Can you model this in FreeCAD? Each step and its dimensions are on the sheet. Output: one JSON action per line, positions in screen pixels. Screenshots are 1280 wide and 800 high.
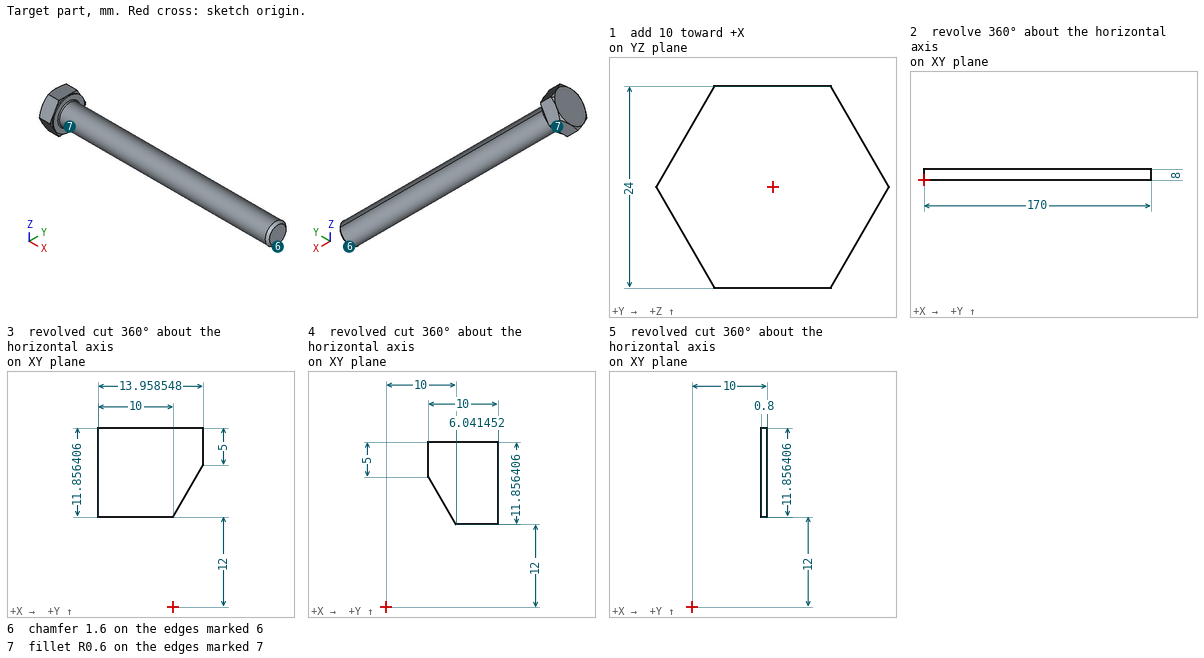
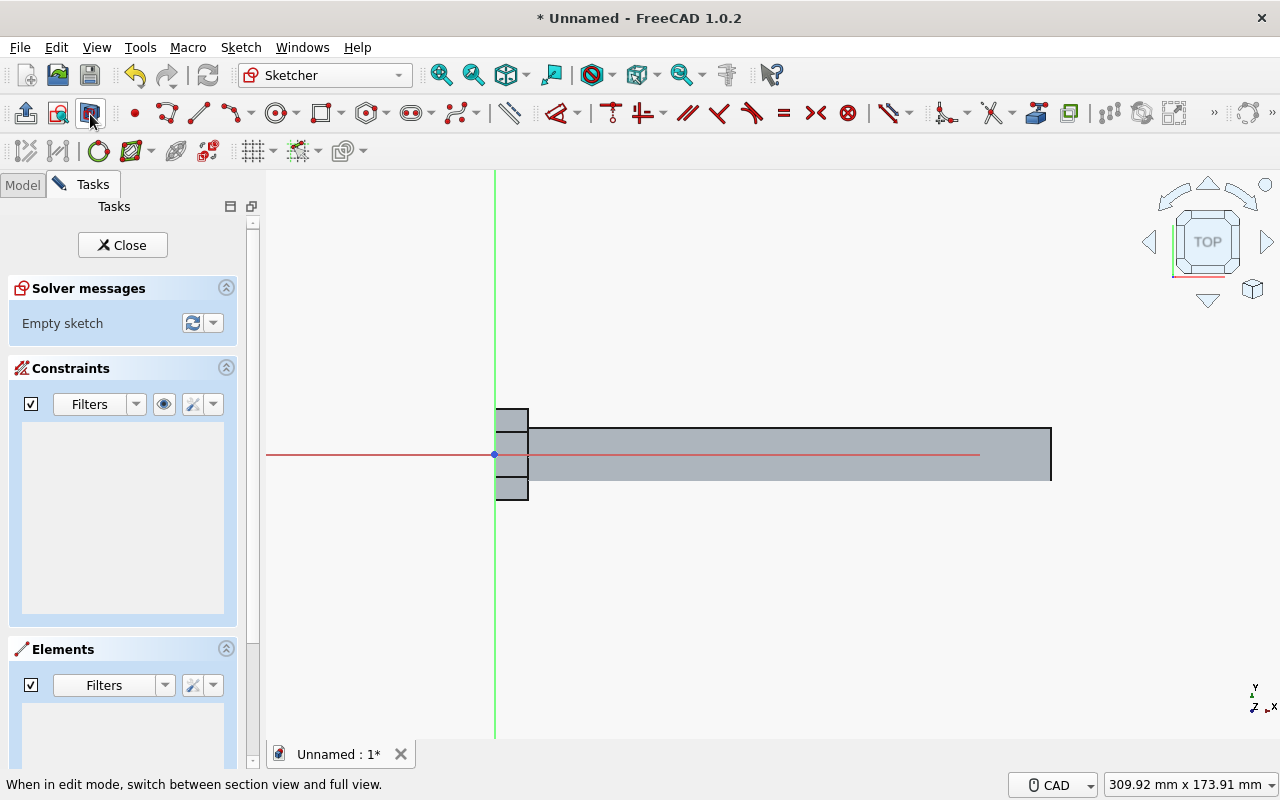
{"action": "scroll", "coordinate": [429, 406], "scroll_direction": "up", "scroll_amount": 8}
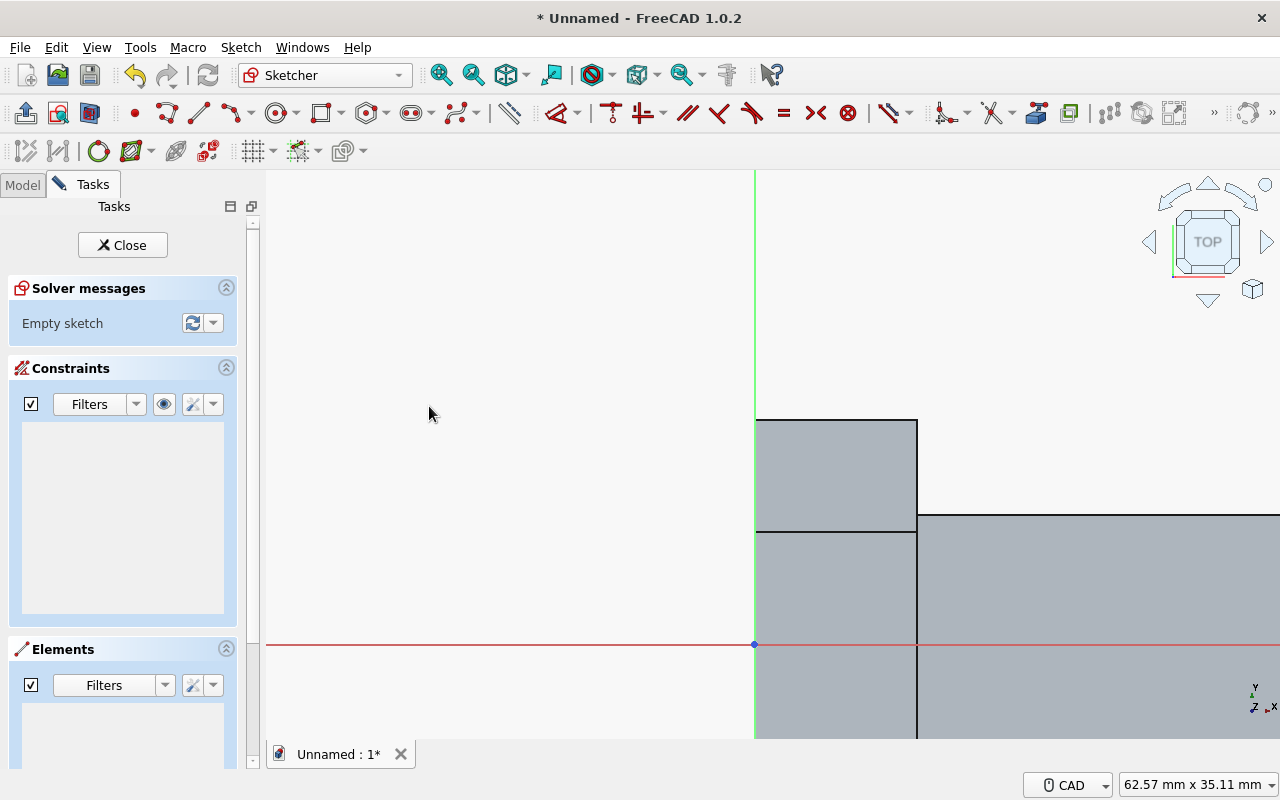
{"action": "left_click", "coordinate": [168, 114]}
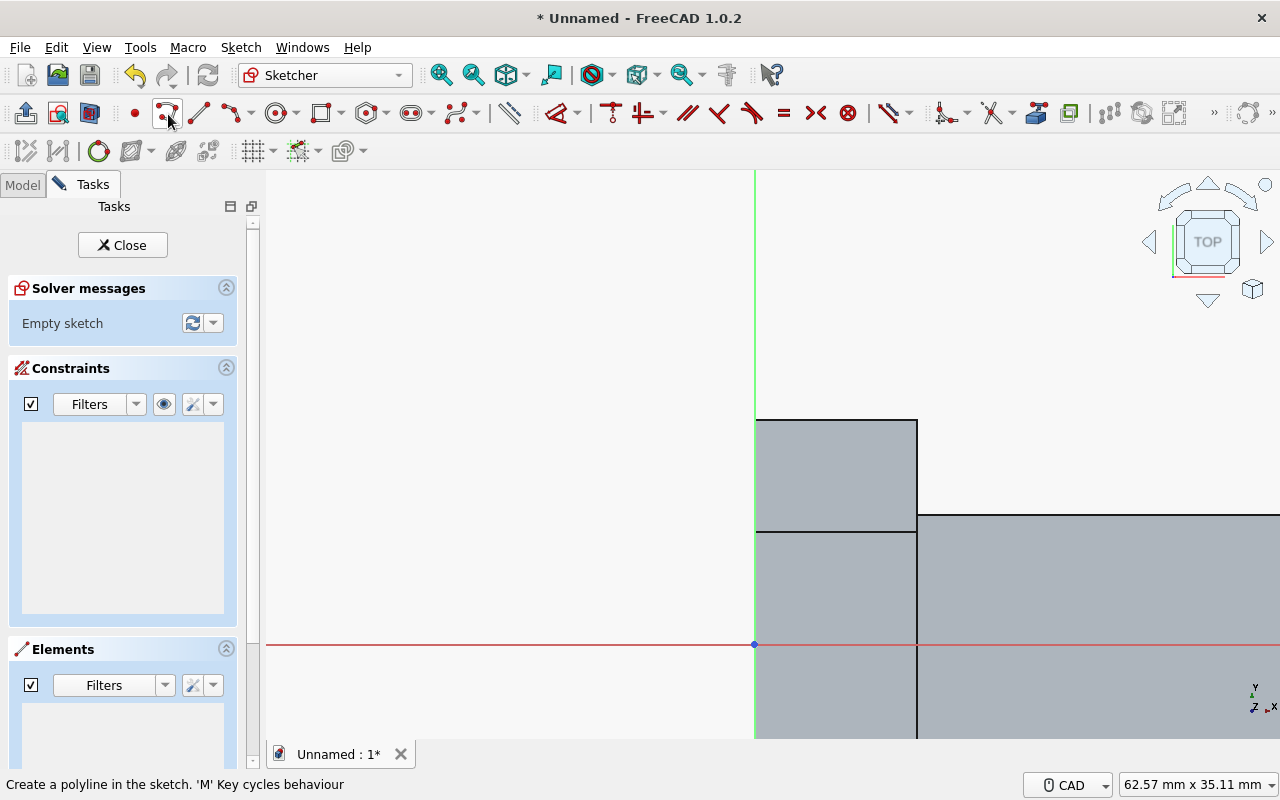
{"action": "left_click", "coordinate": [755, 450]}
{"action": "left_click", "coordinate": [819, 339]}
{"action": "left_click", "coordinate": [819, 258]}
{"action": "left_click", "coordinate": [593, 258]}
{"action": "left_click", "coordinate": [593, 450]}
{"action": "left_click", "coordinate": [755, 451]}
{"action": "key", "text": "Escape"}
{"action": "key", "text": "Escape"}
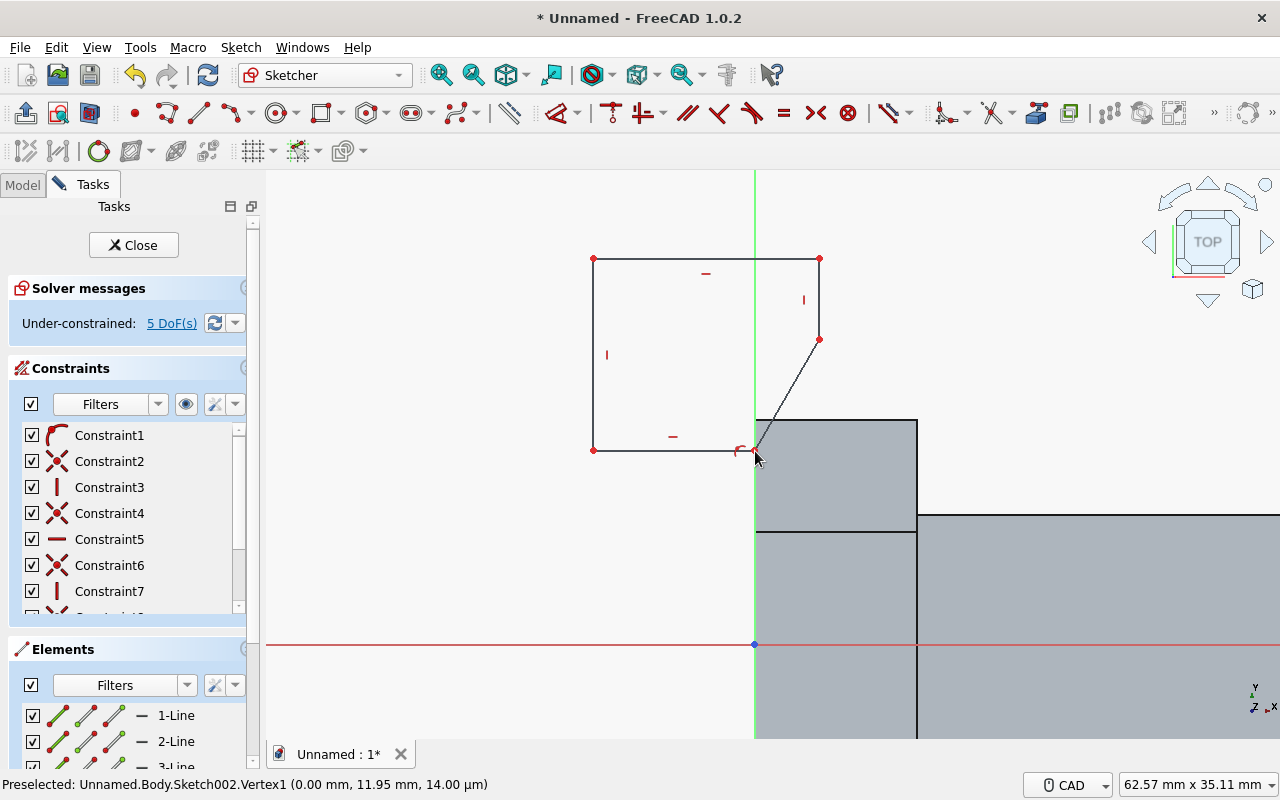
{"action": "left_click", "coordinate": [556, 114]}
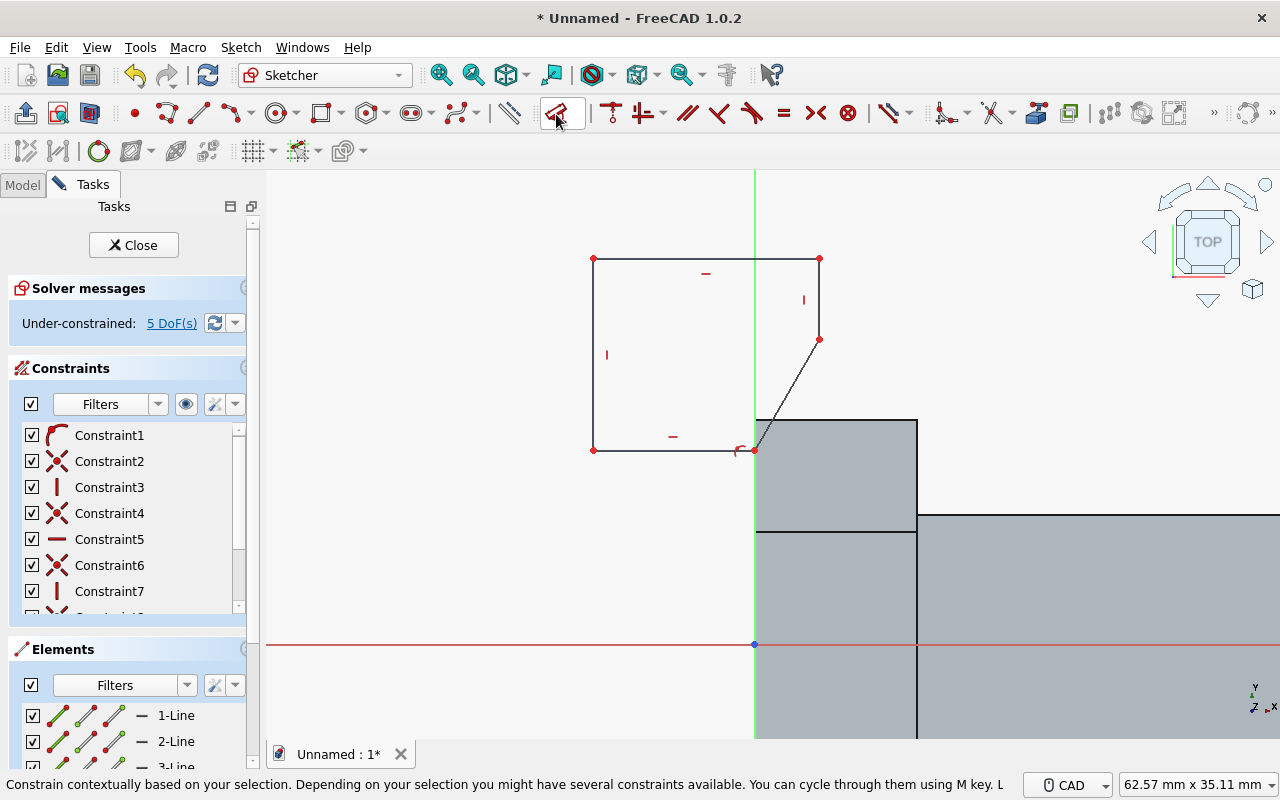
{"action": "left_click", "coordinate": [819, 316]}
{"action": "left_click", "coordinate": [853, 299]}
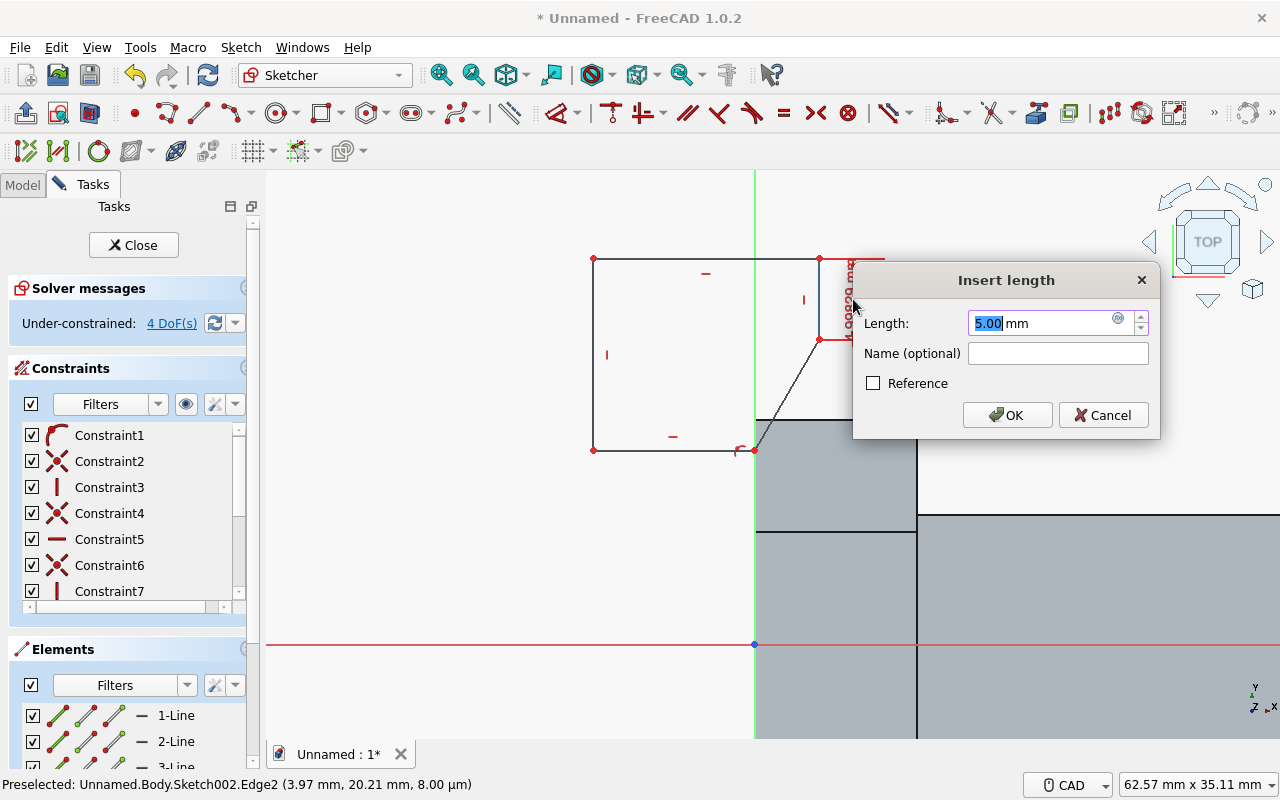
{"action": "type", "text": "5"}
{"action": "key", "text": "Return"}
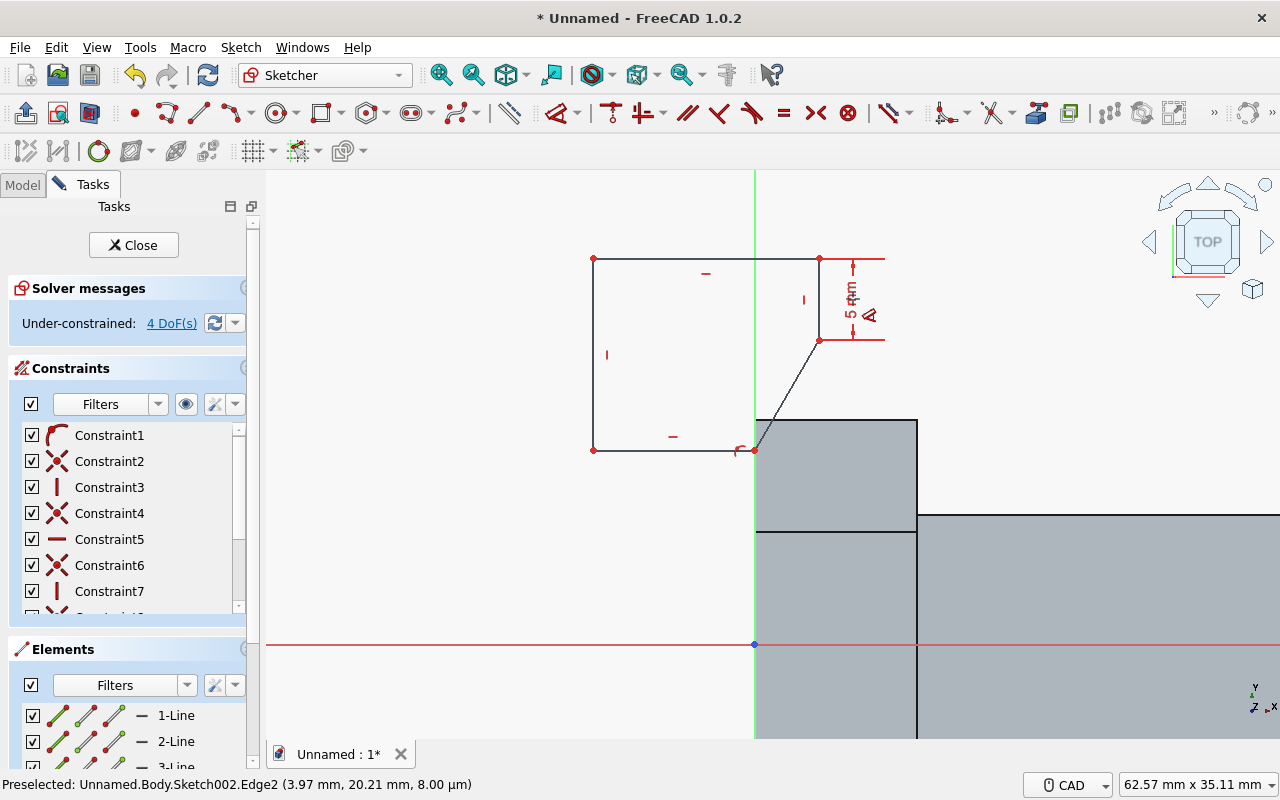
{"action": "left_click", "coordinate": [642, 451]}
{"action": "left_click", "coordinate": [674, 417]}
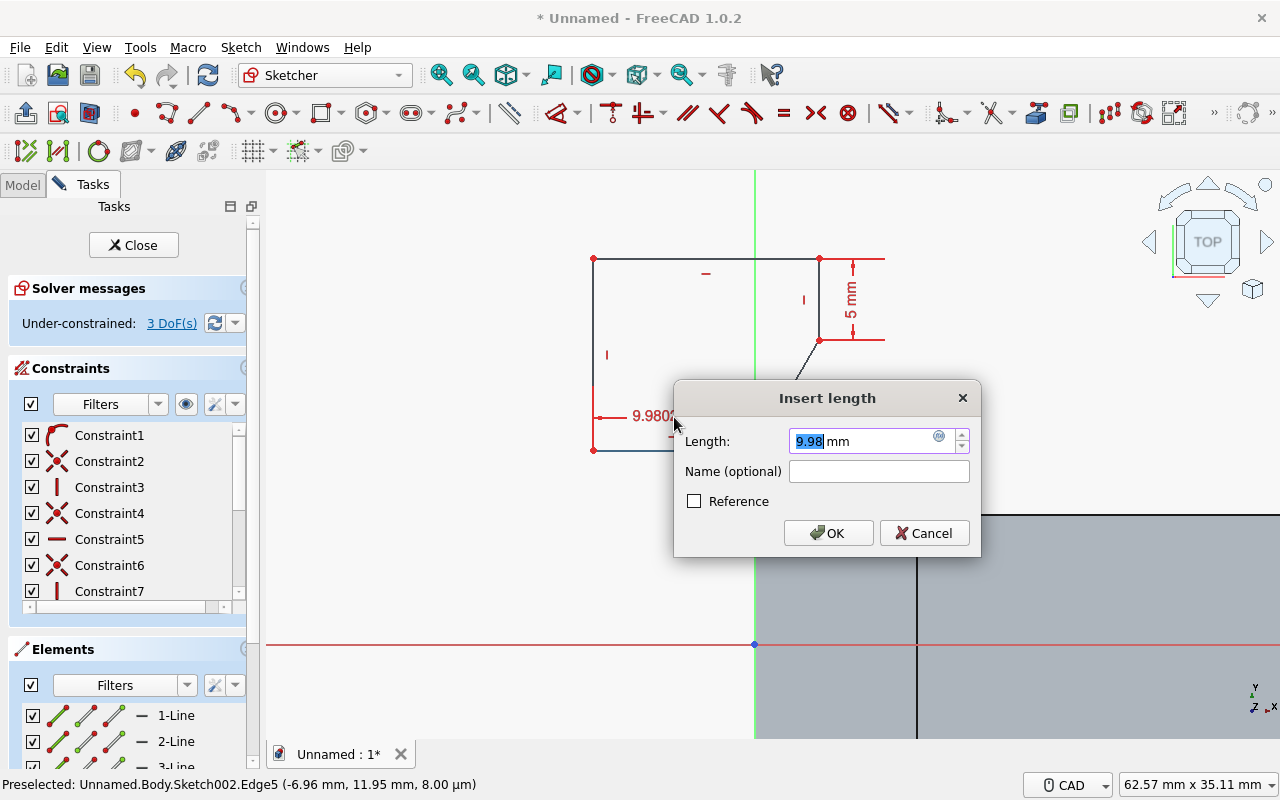
{"action": "type", "text": "10"}
{"action": "key", "text": "Return"}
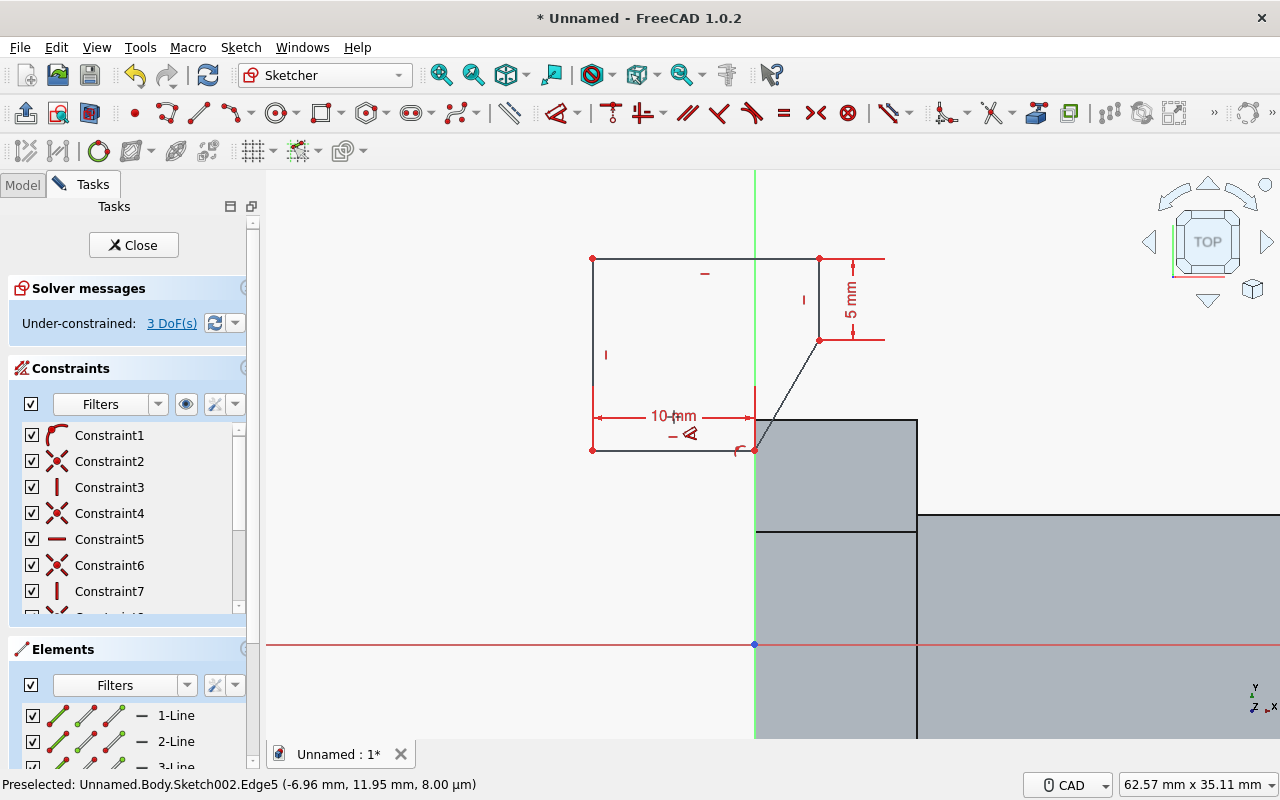
{"action": "left_click", "coordinate": [755, 451]}
{"action": "left_click", "coordinate": [789, 548]}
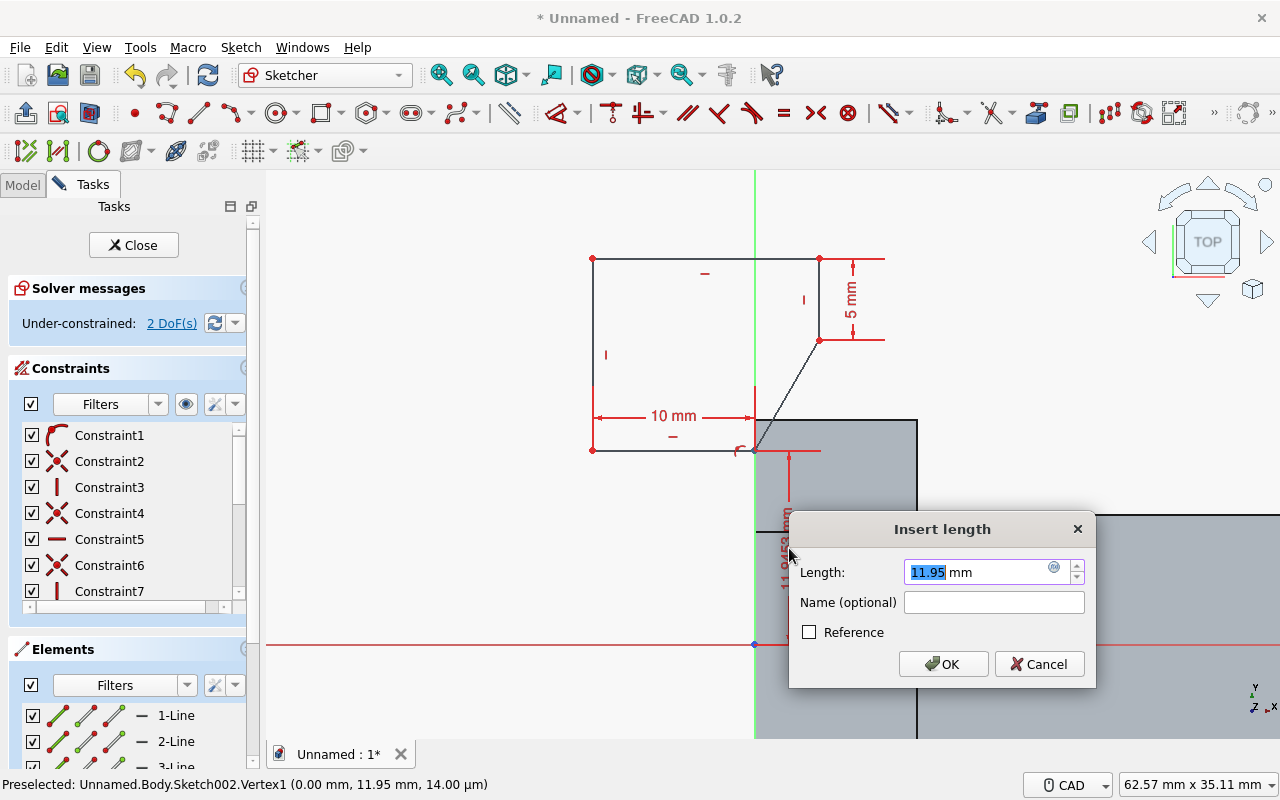
{"action": "type", "text": "12"}
{"action": "key", "text": "Return"}